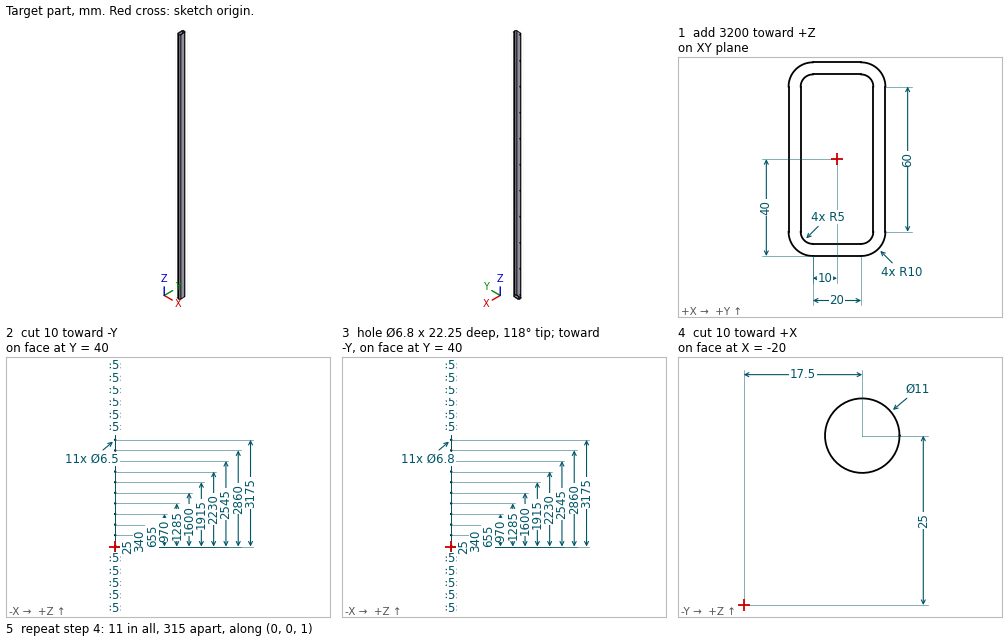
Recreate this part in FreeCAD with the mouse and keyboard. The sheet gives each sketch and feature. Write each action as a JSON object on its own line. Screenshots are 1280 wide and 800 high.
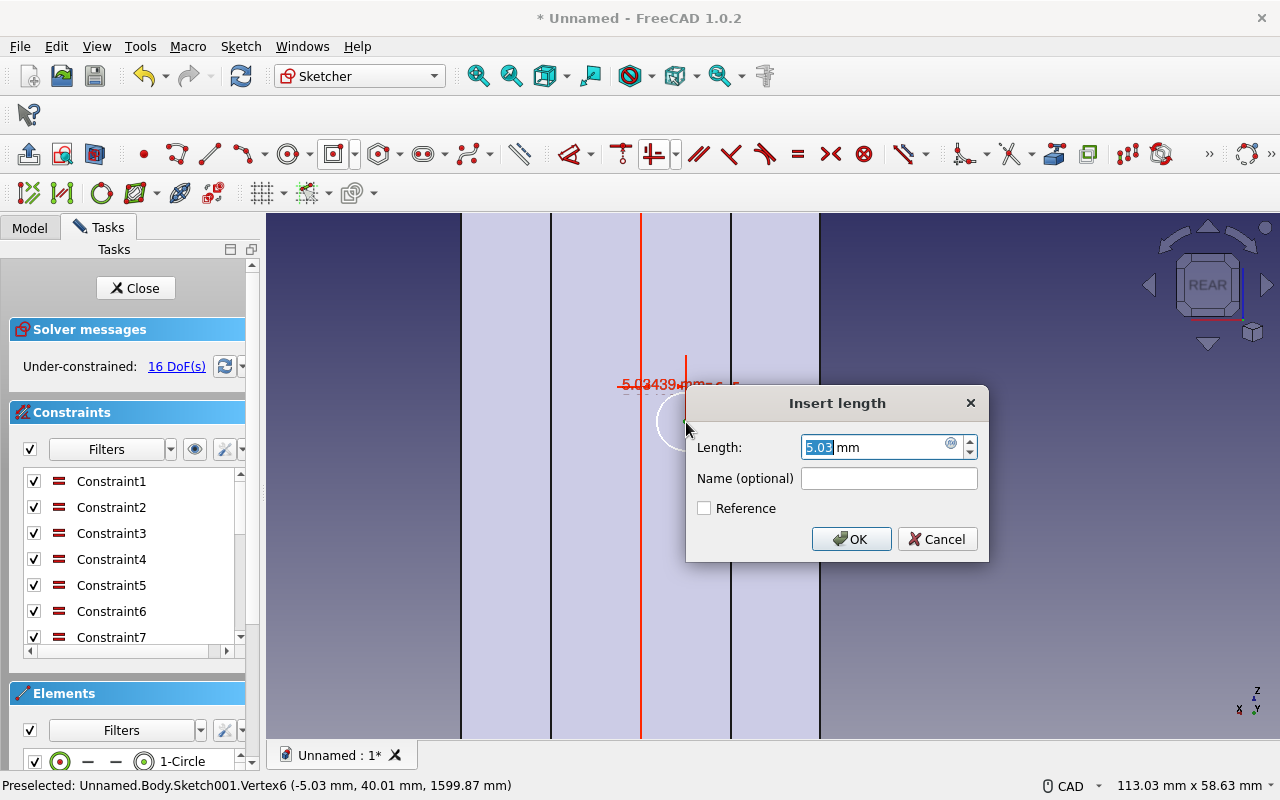
{"action": "type", "text": "5"}
{"action": "key", "text": "Return"}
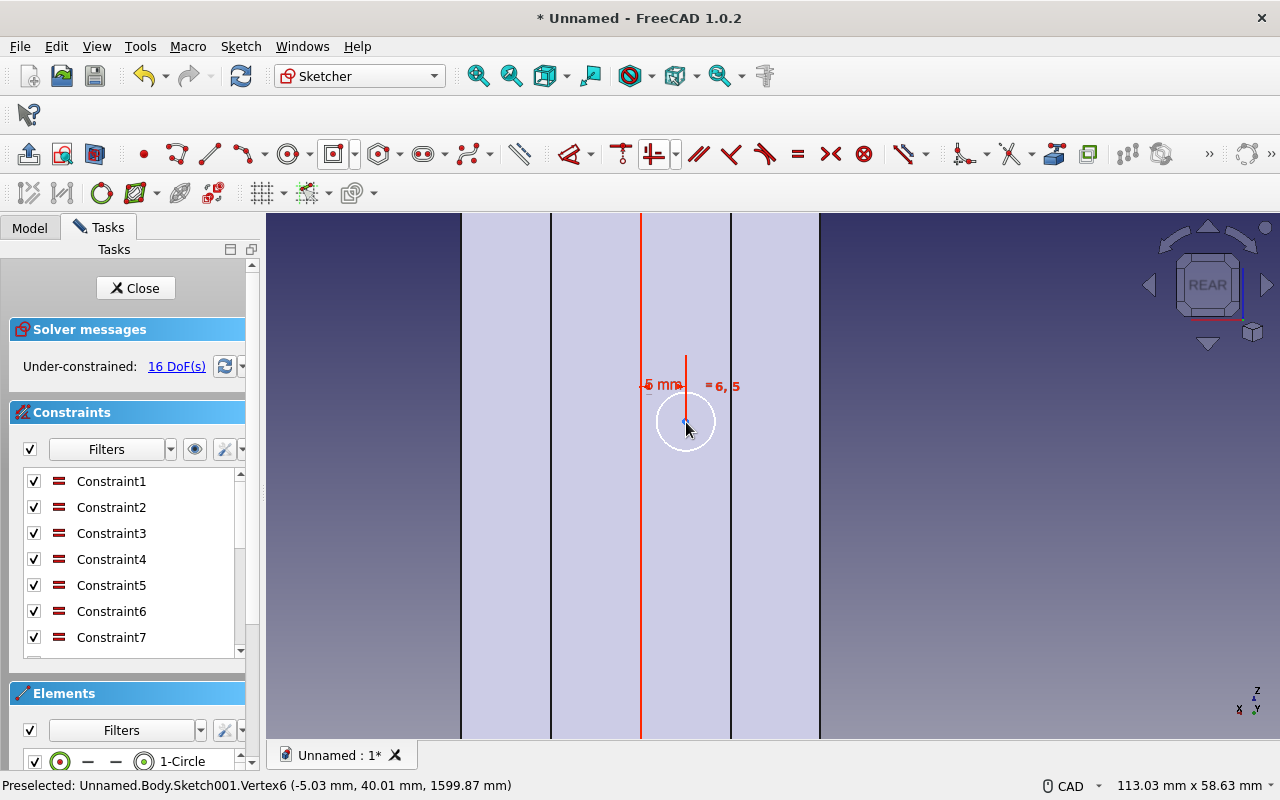
{"action": "scroll", "coordinate": [704, 476], "scroll_direction": "down", "scroll_amount": 15}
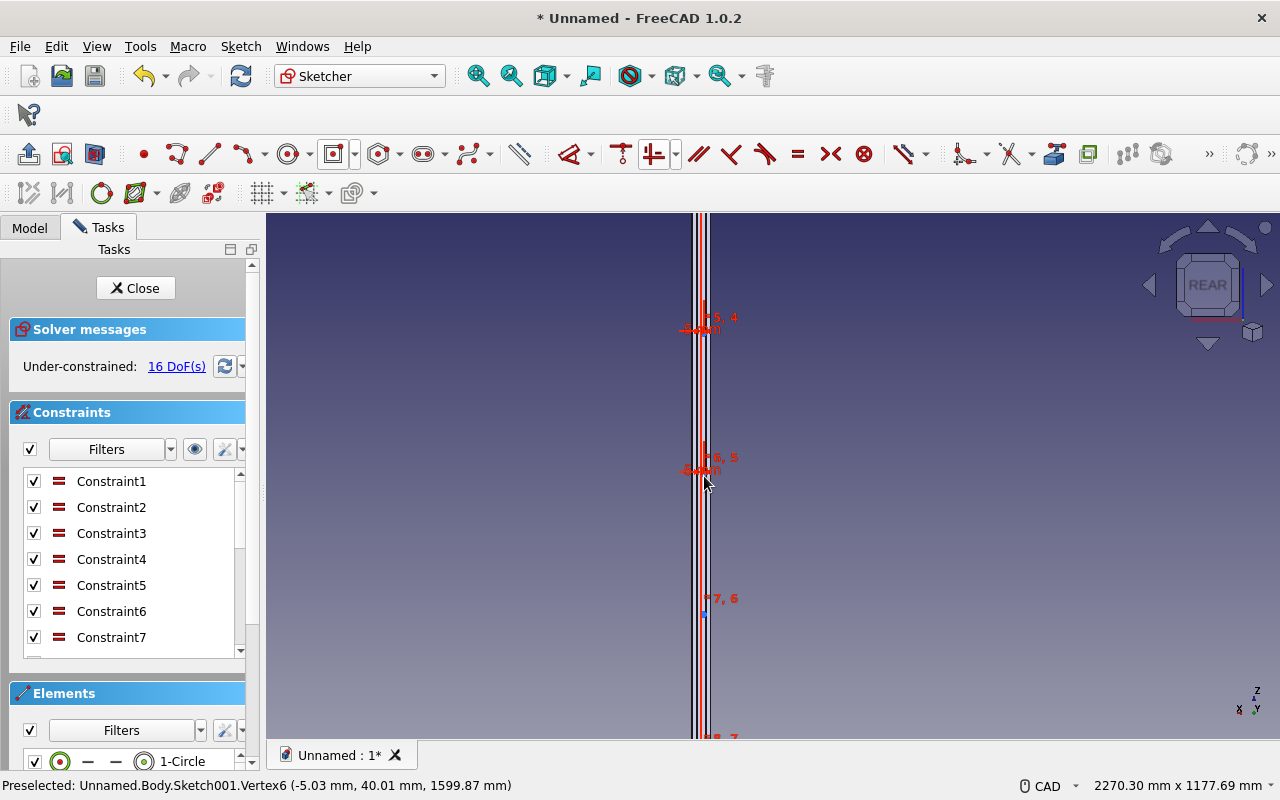
{"action": "scroll", "coordinate": [705, 475], "scroll_direction": "down", "scroll_amount": 7}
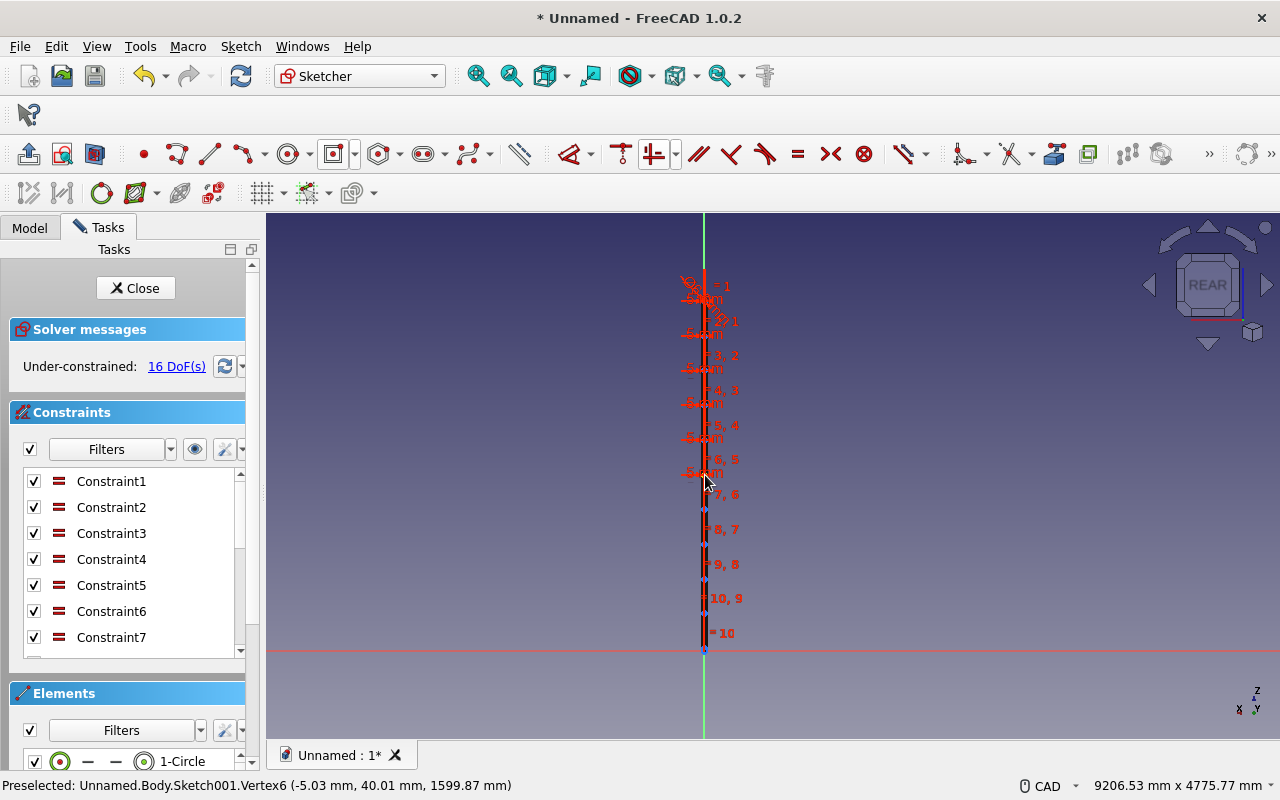
{"action": "scroll", "coordinate": [705, 510], "scroll_direction": "up", "scroll_amount": 22}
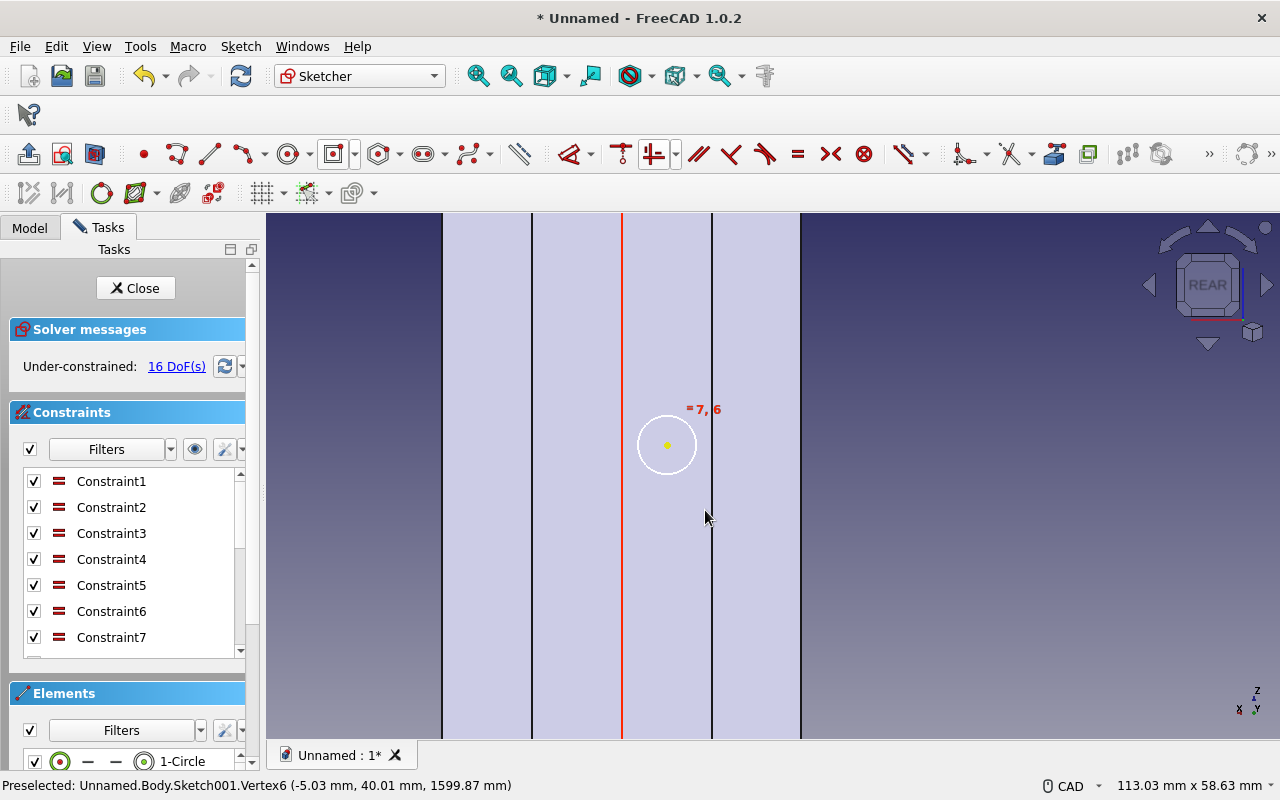
{"action": "left_click", "coordinate": [667, 445]}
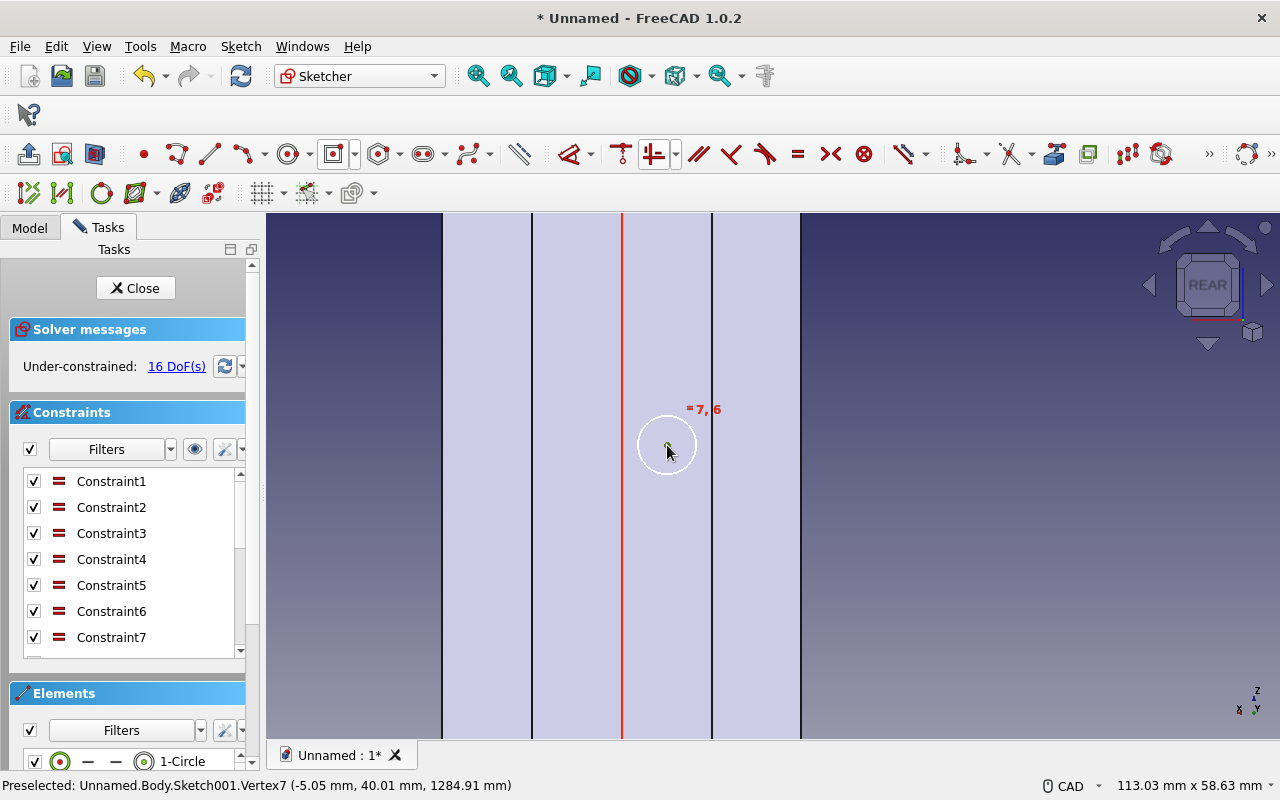
{"action": "key", "text": "l"}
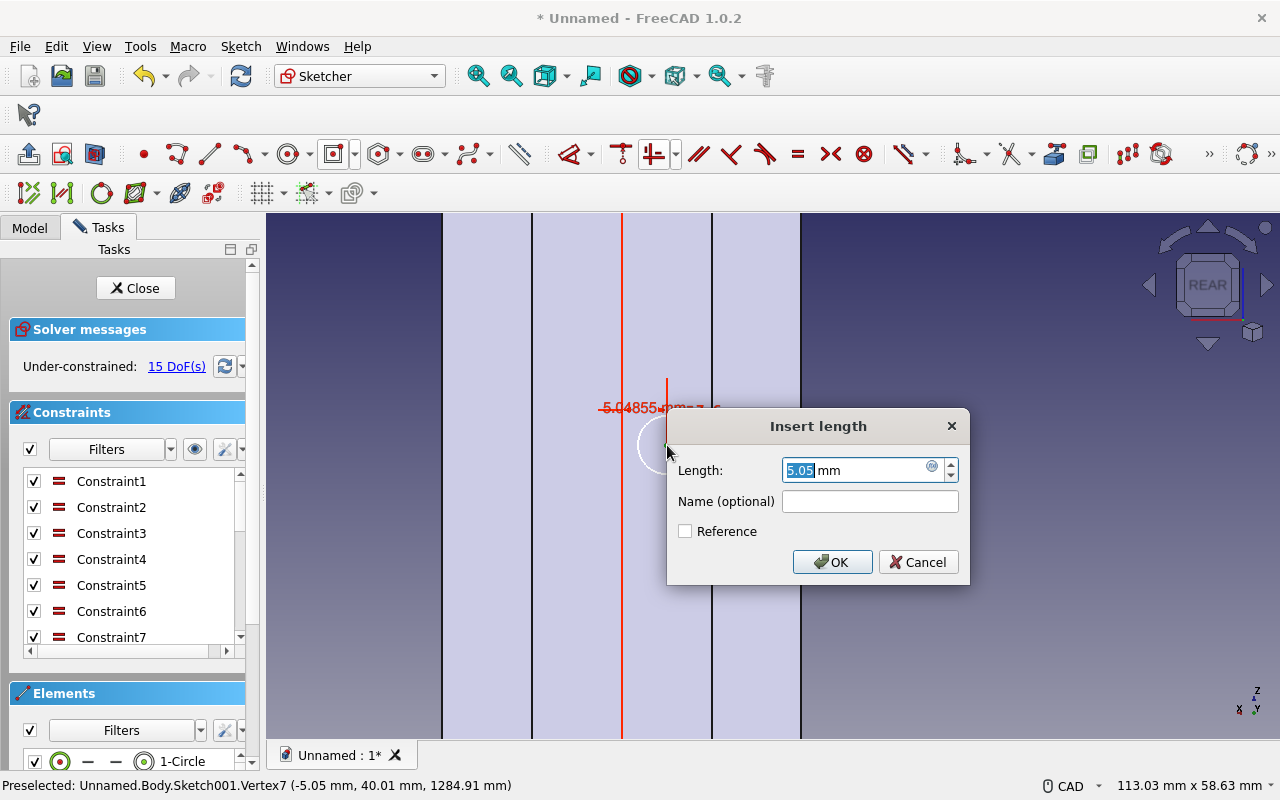
{"action": "type", "text": "5"}
{"action": "key", "text": "Return"}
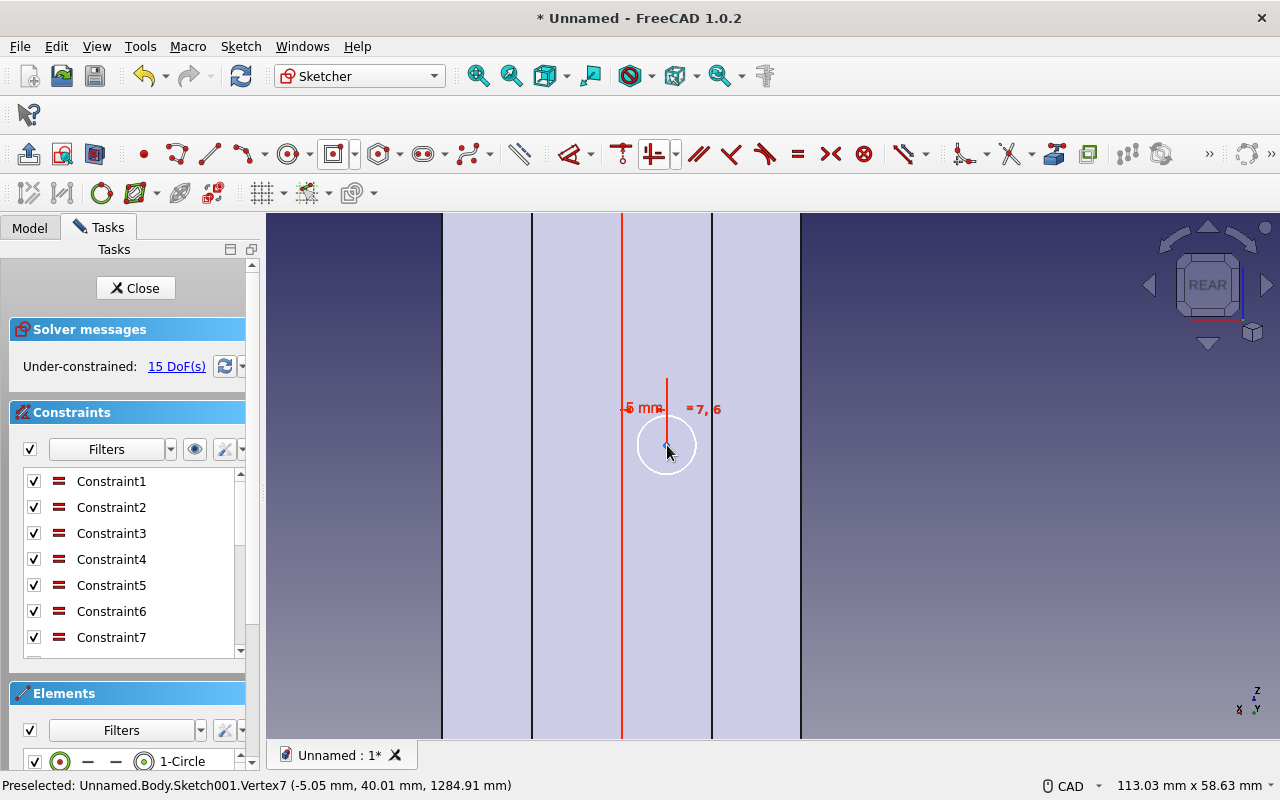
{"action": "scroll", "coordinate": [704, 476], "scroll_direction": "down", "scroll_amount": 15}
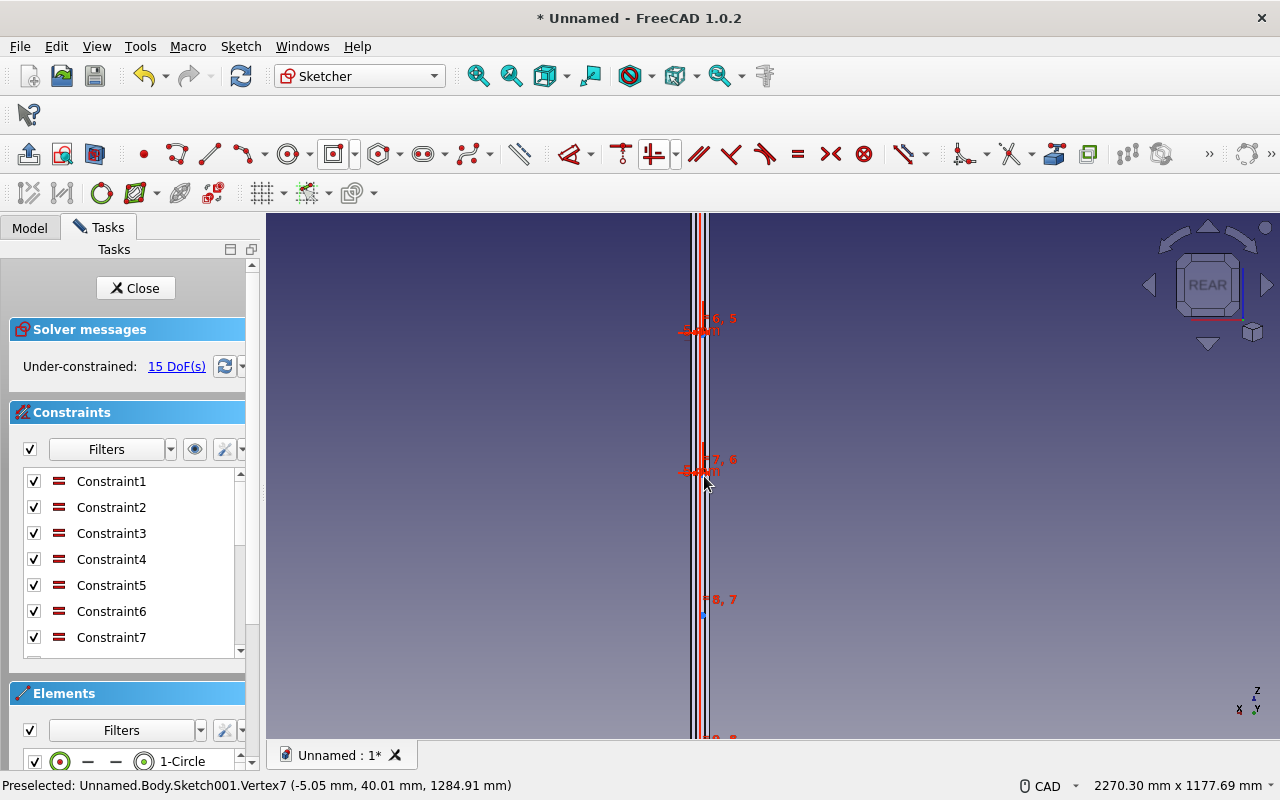
{"action": "scroll", "coordinate": [705, 521], "scroll_direction": "down", "scroll_amount": 7}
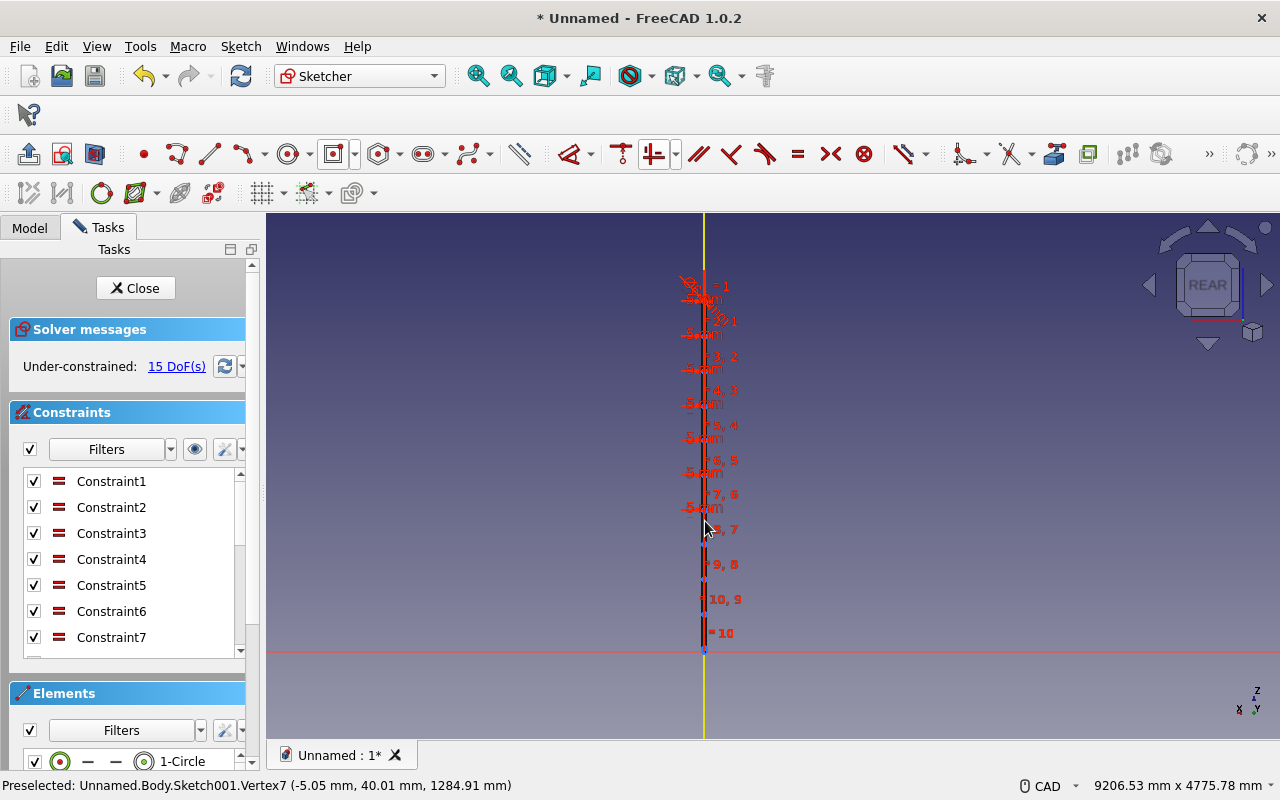
{"action": "scroll", "coordinate": [705, 545], "scroll_direction": "up", "scroll_amount": 22}